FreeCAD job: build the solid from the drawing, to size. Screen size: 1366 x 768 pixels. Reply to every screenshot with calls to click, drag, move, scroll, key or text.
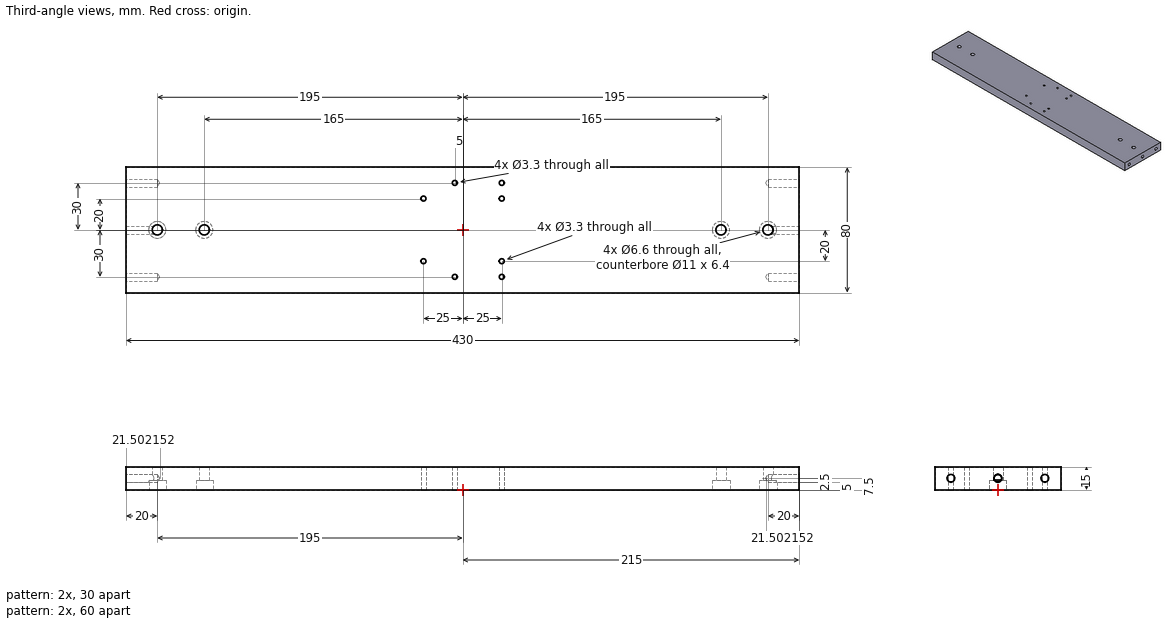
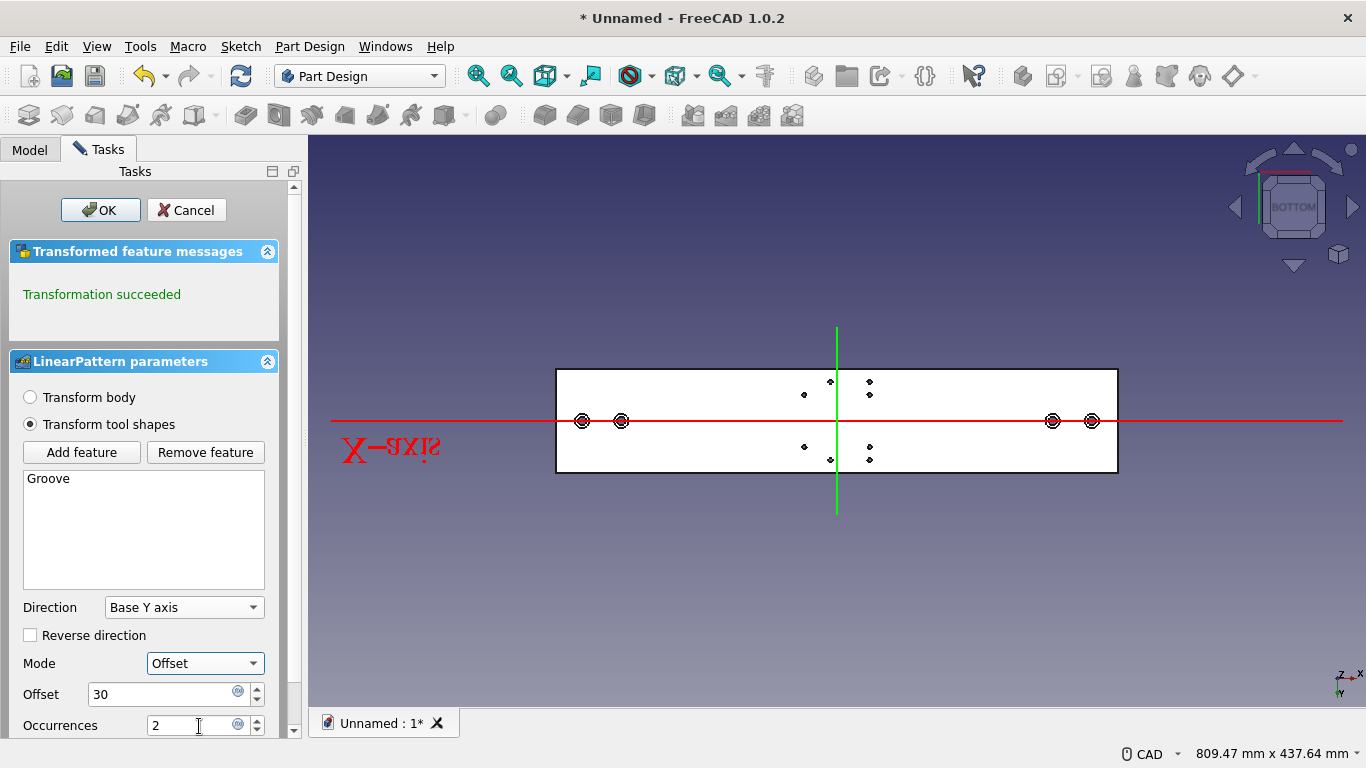
click(31, 635)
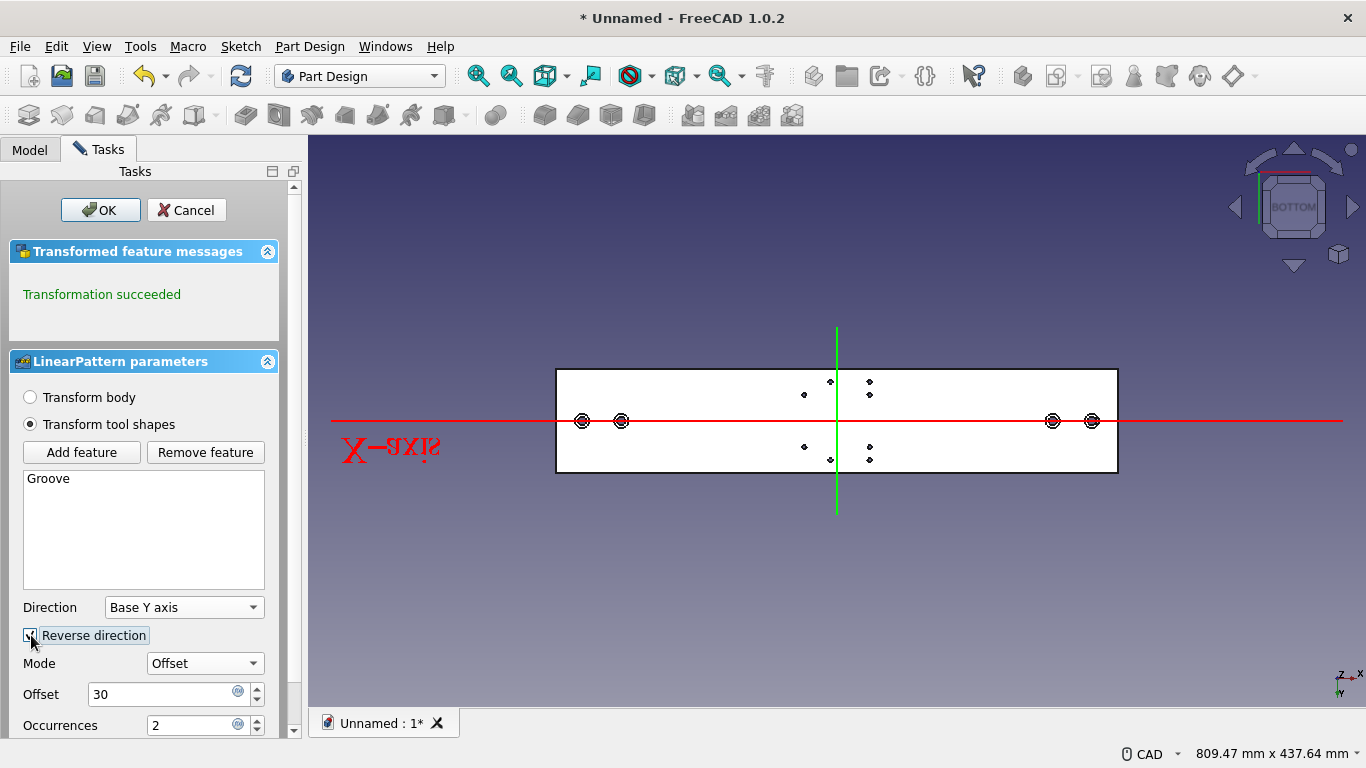
click(101, 210)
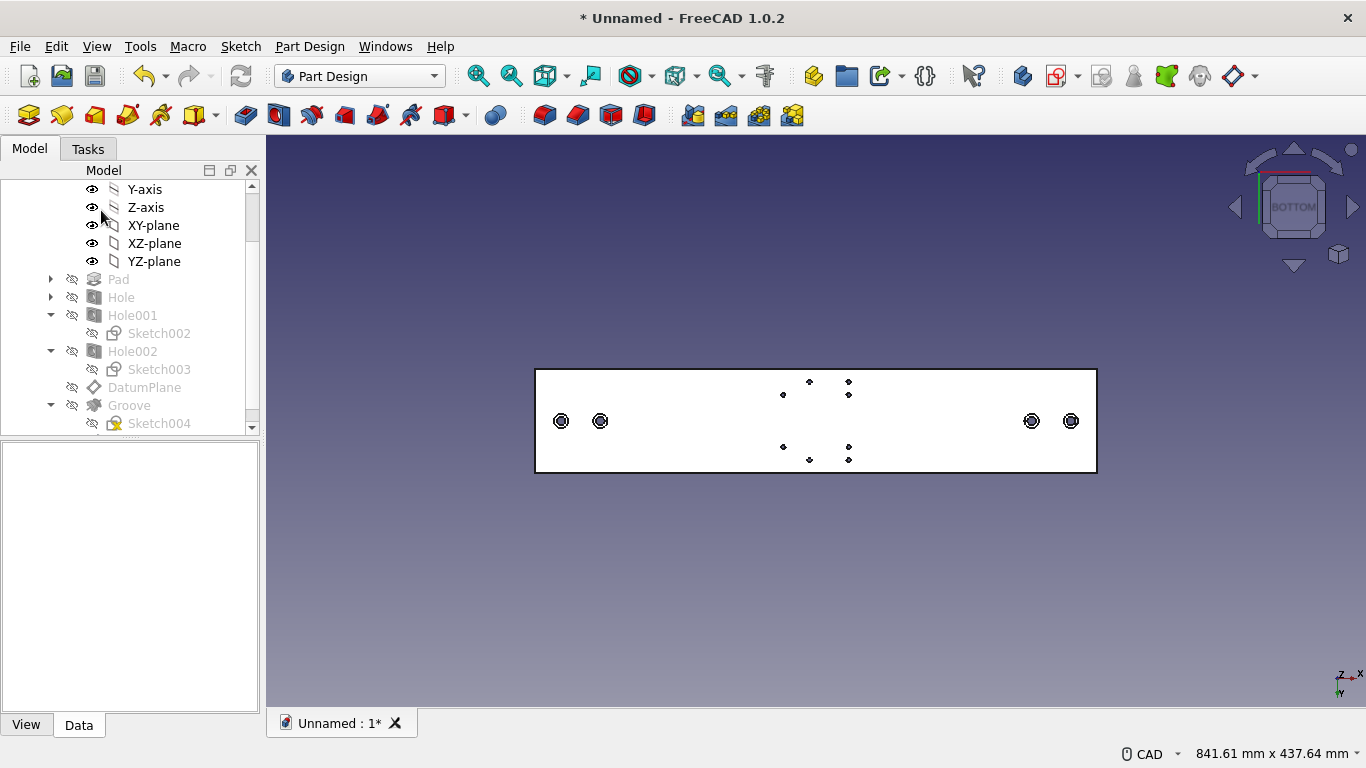
click(117, 405)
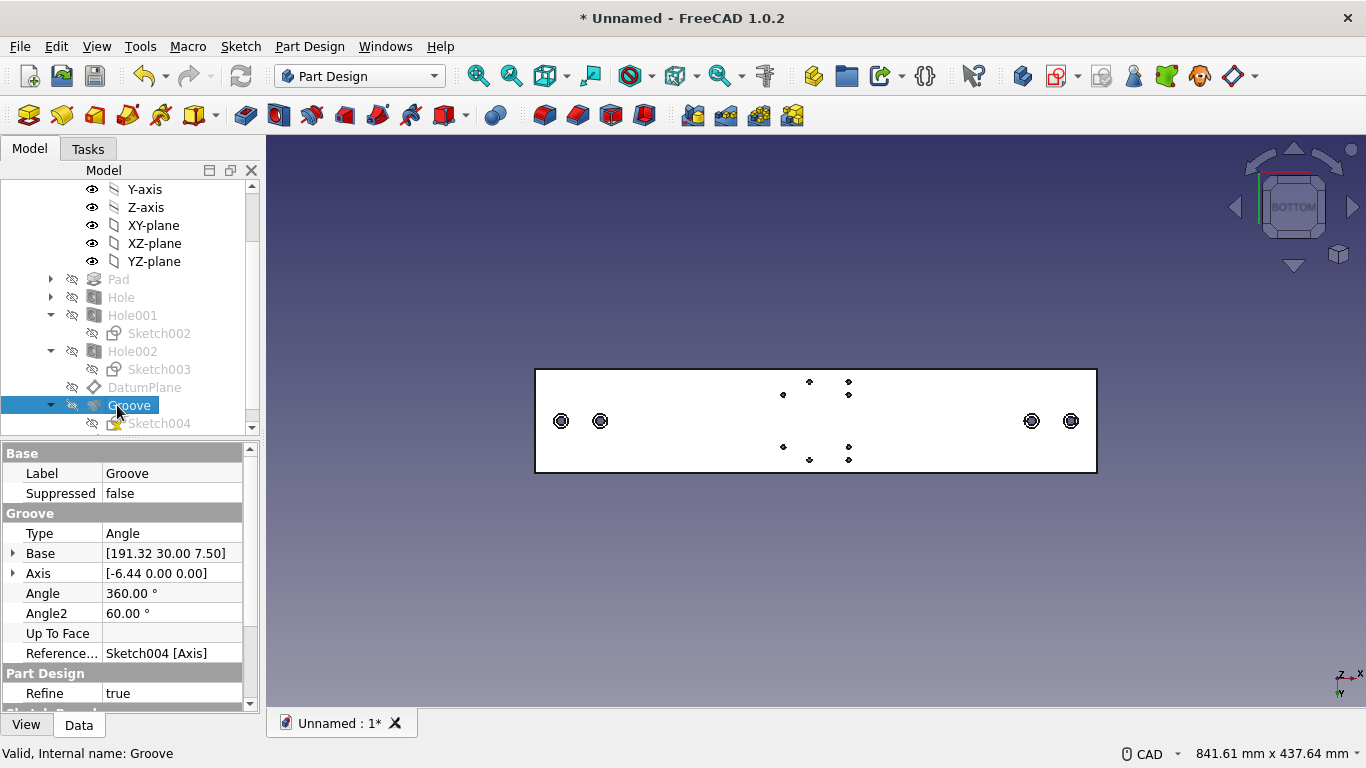
click(726, 116)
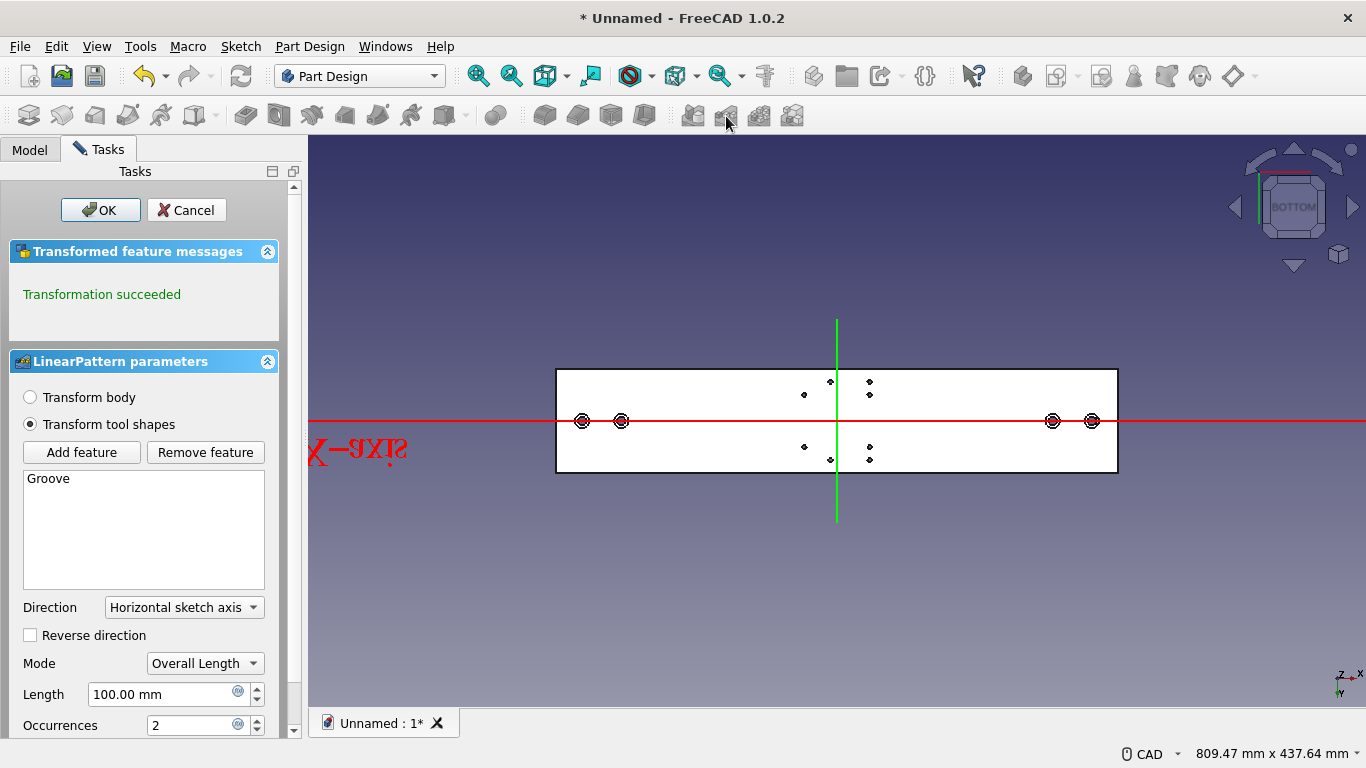
click(185, 608)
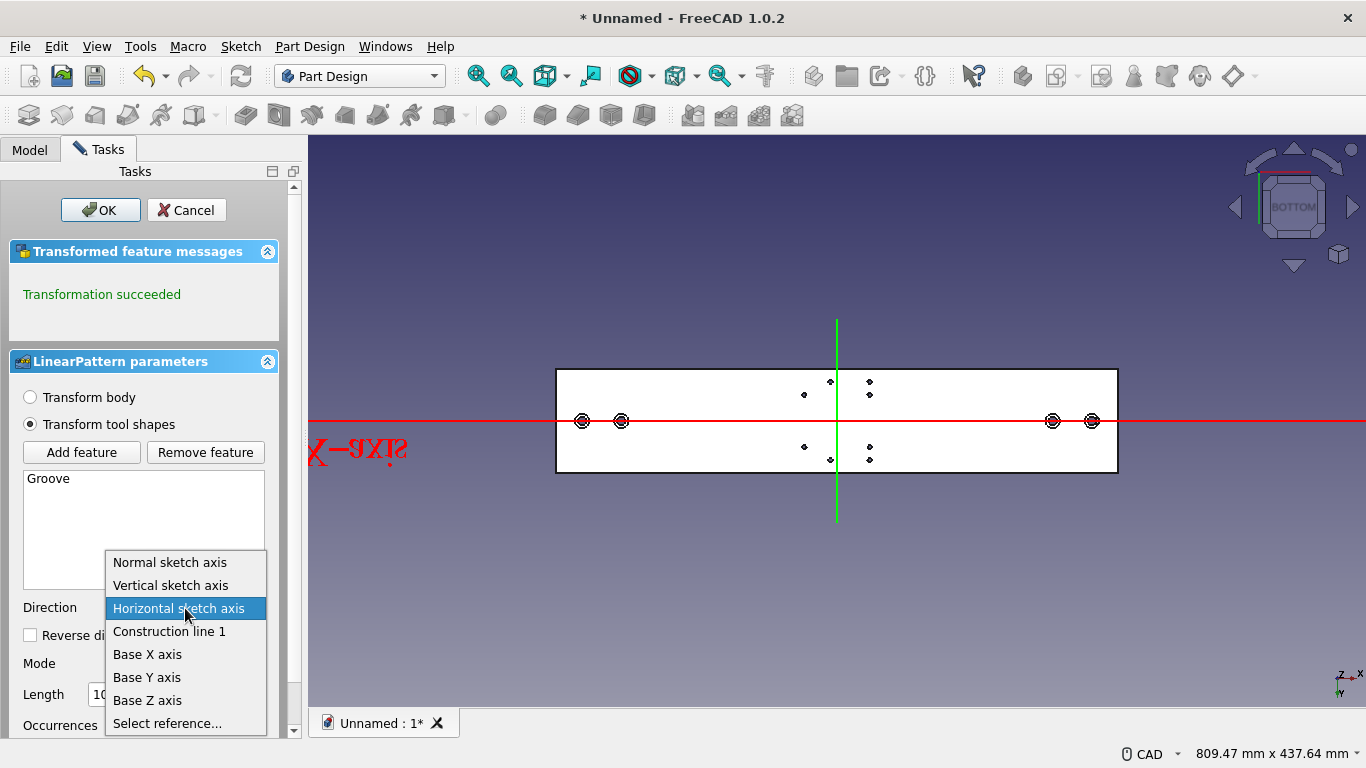
click(184, 678)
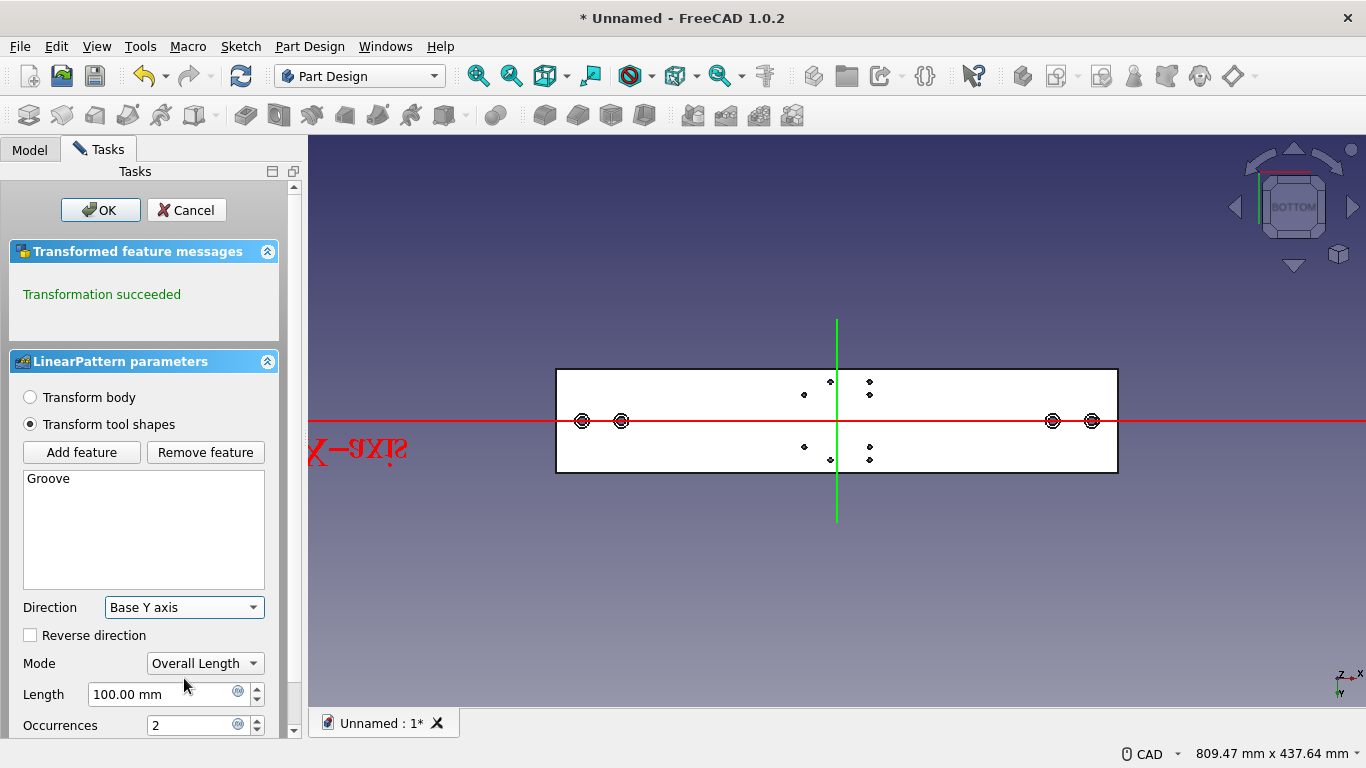
click(206, 664)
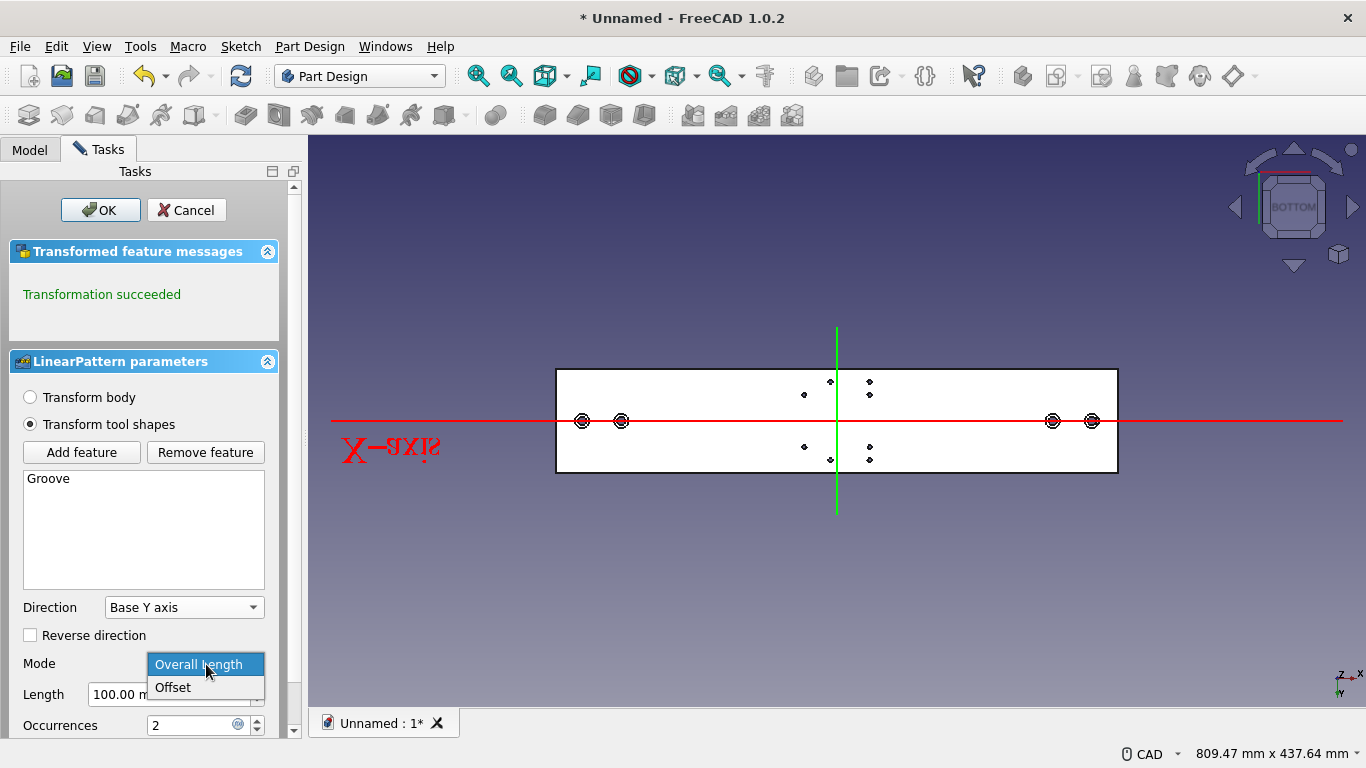
click(204, 688)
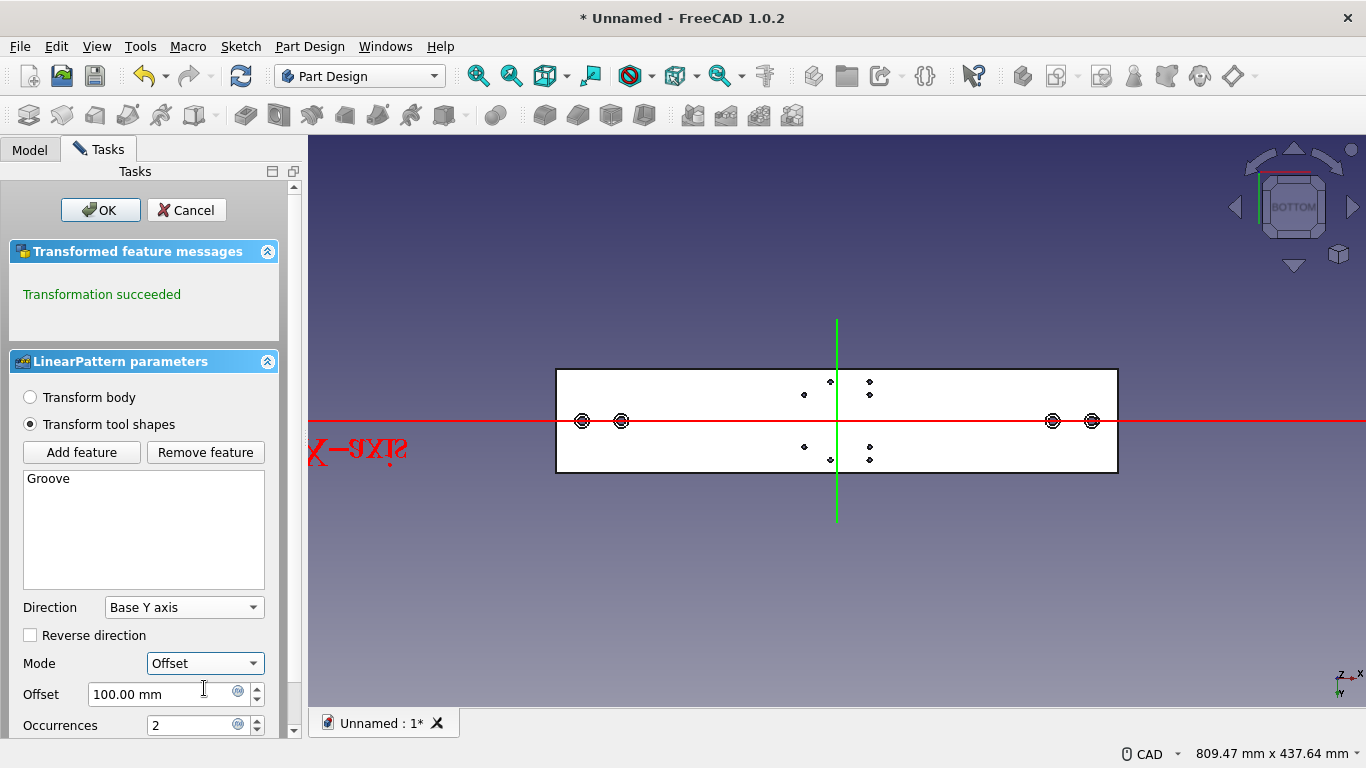
triple_click(170, 694)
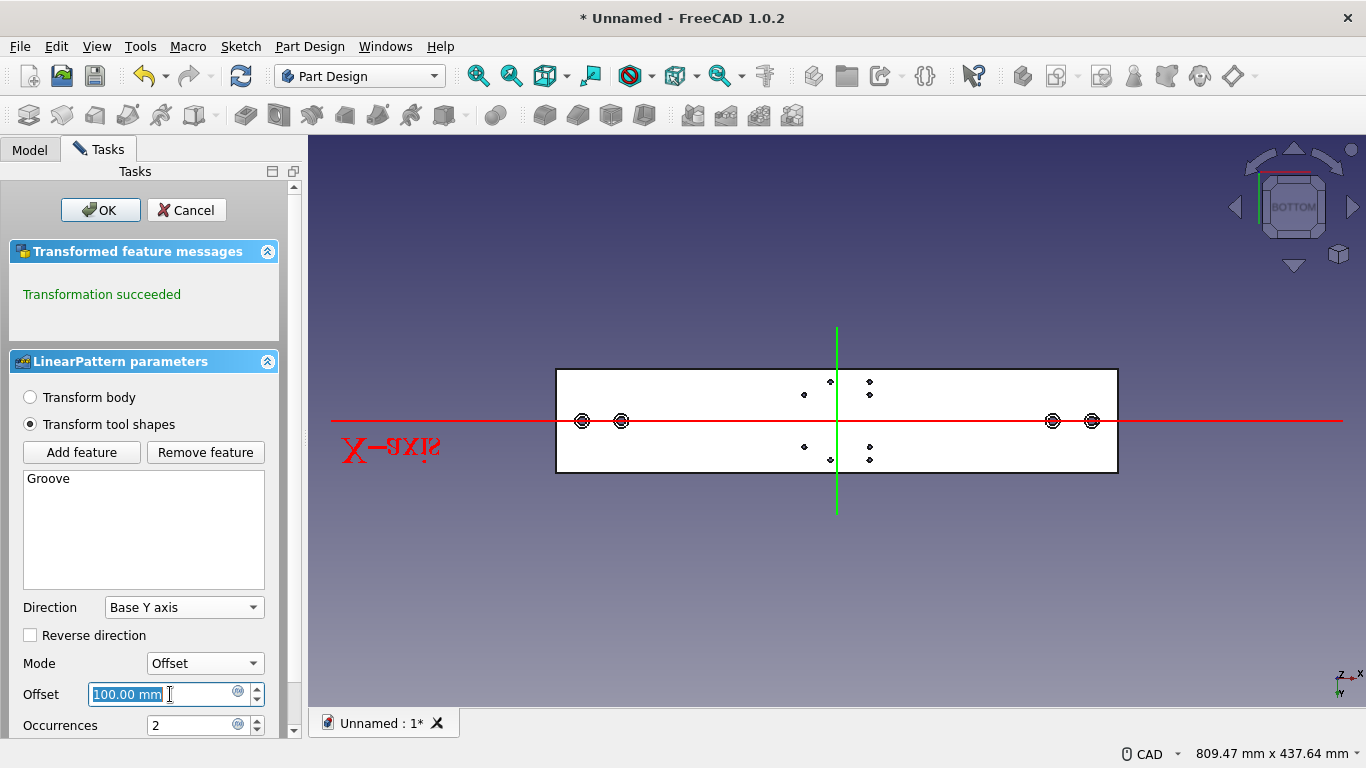
text(60)
key(Tab)